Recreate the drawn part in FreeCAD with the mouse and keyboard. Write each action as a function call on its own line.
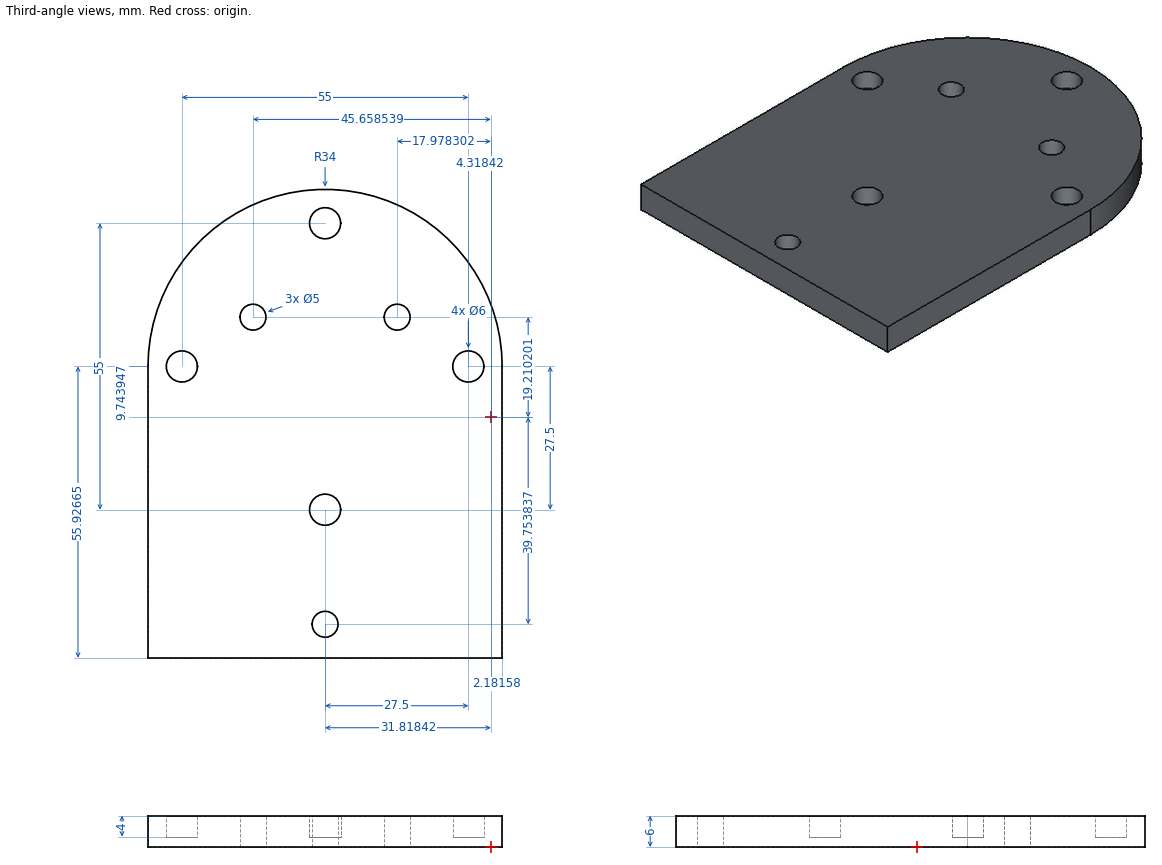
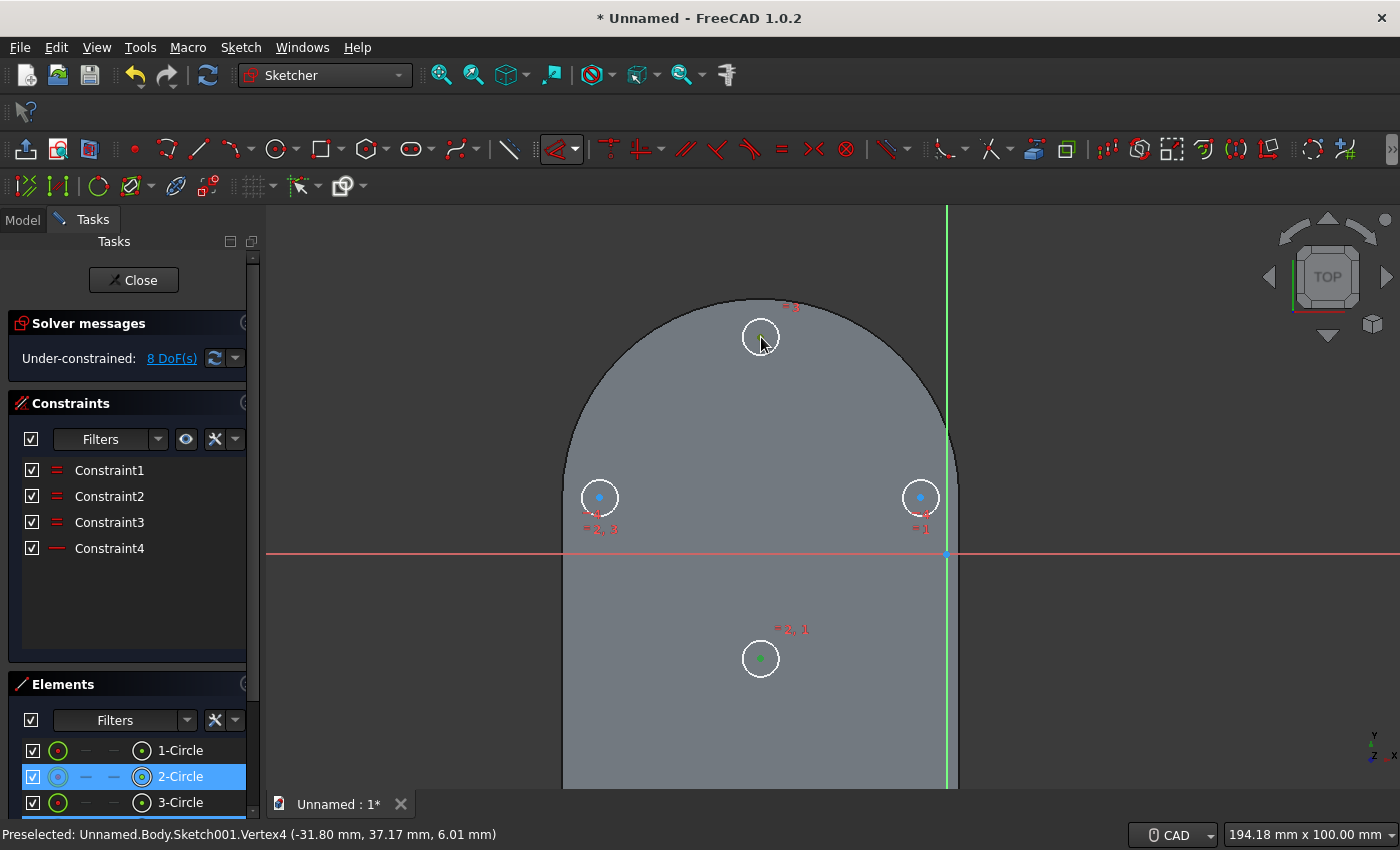
key(v)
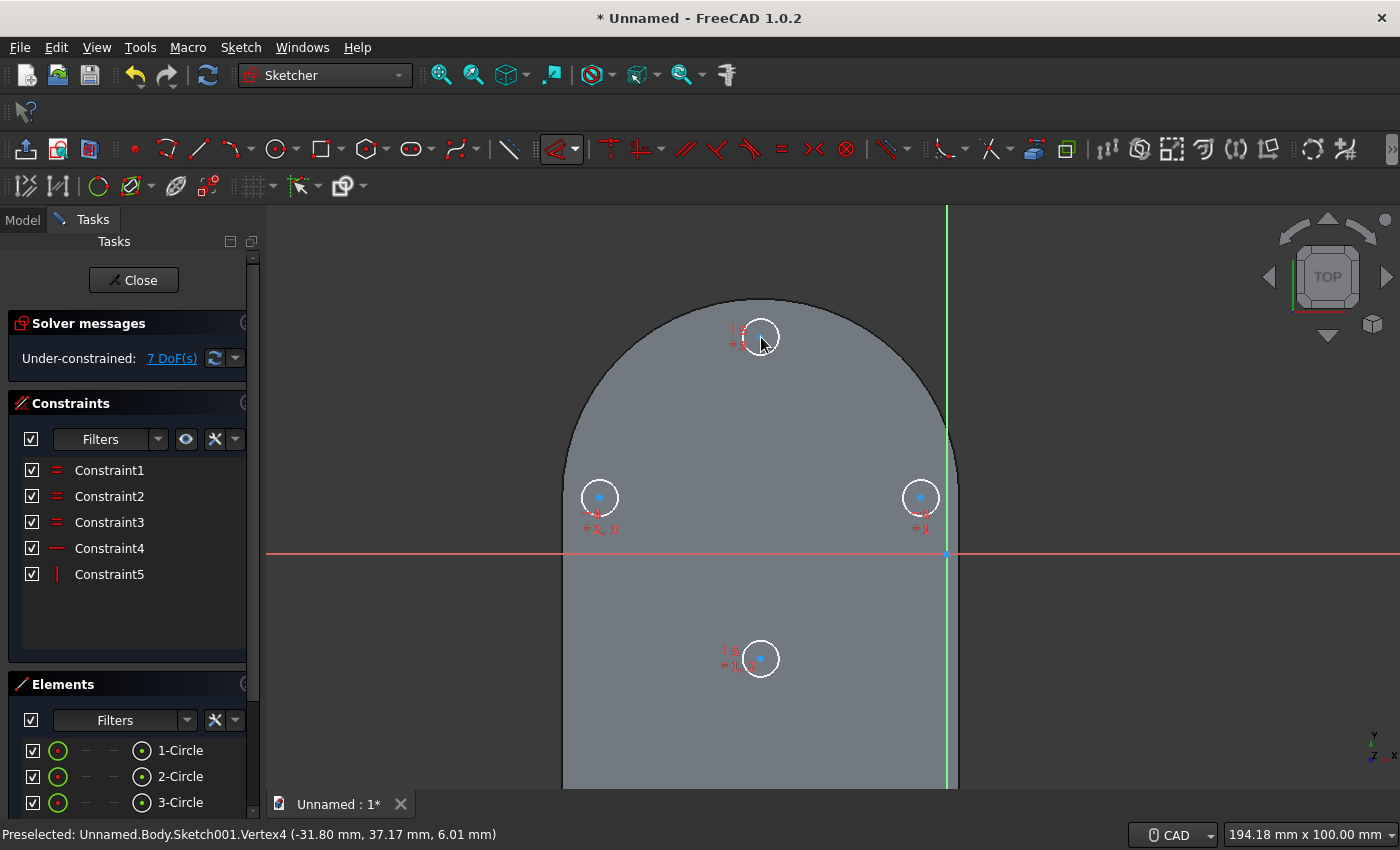
click(934, 485)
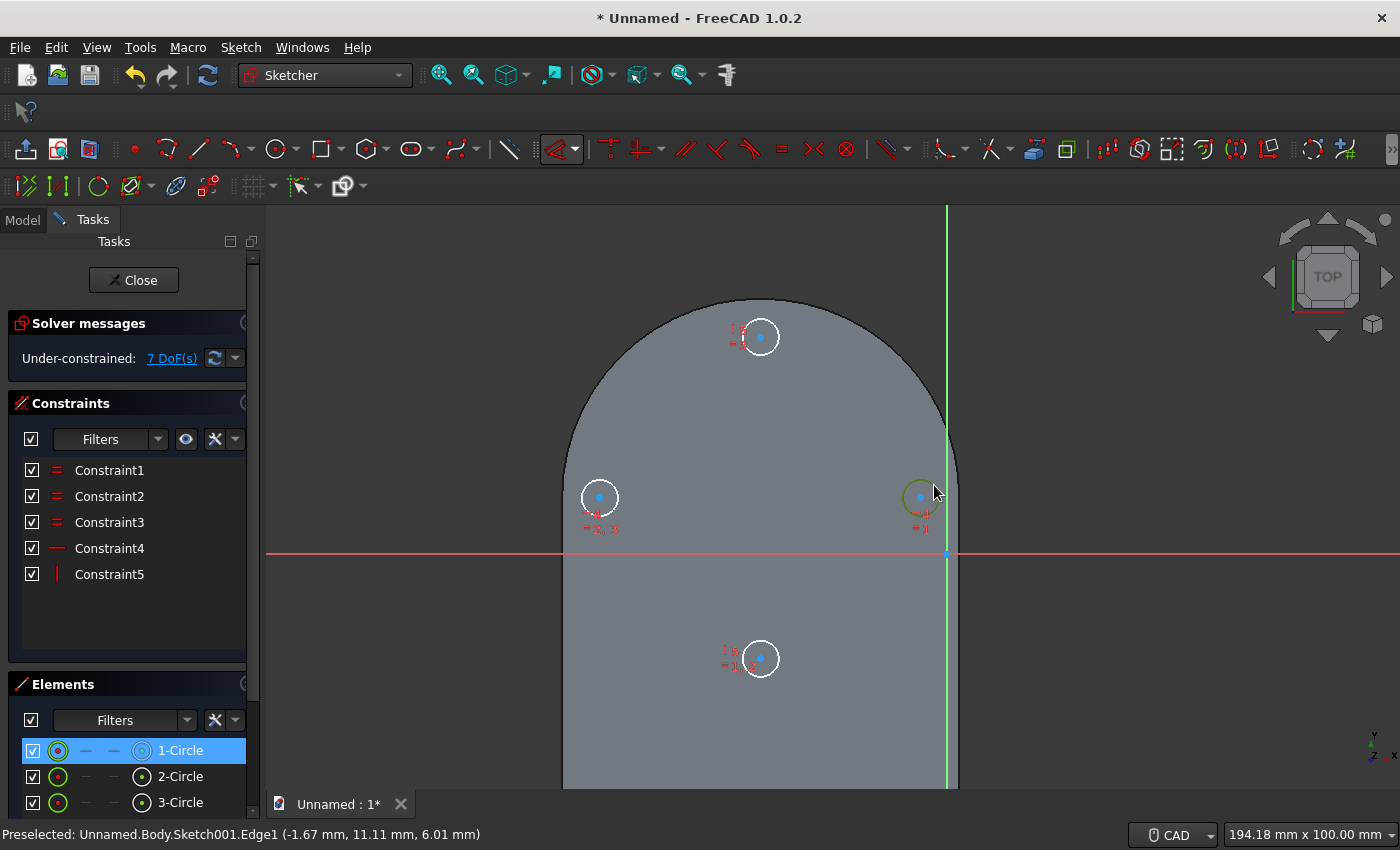
key(k)
key(o)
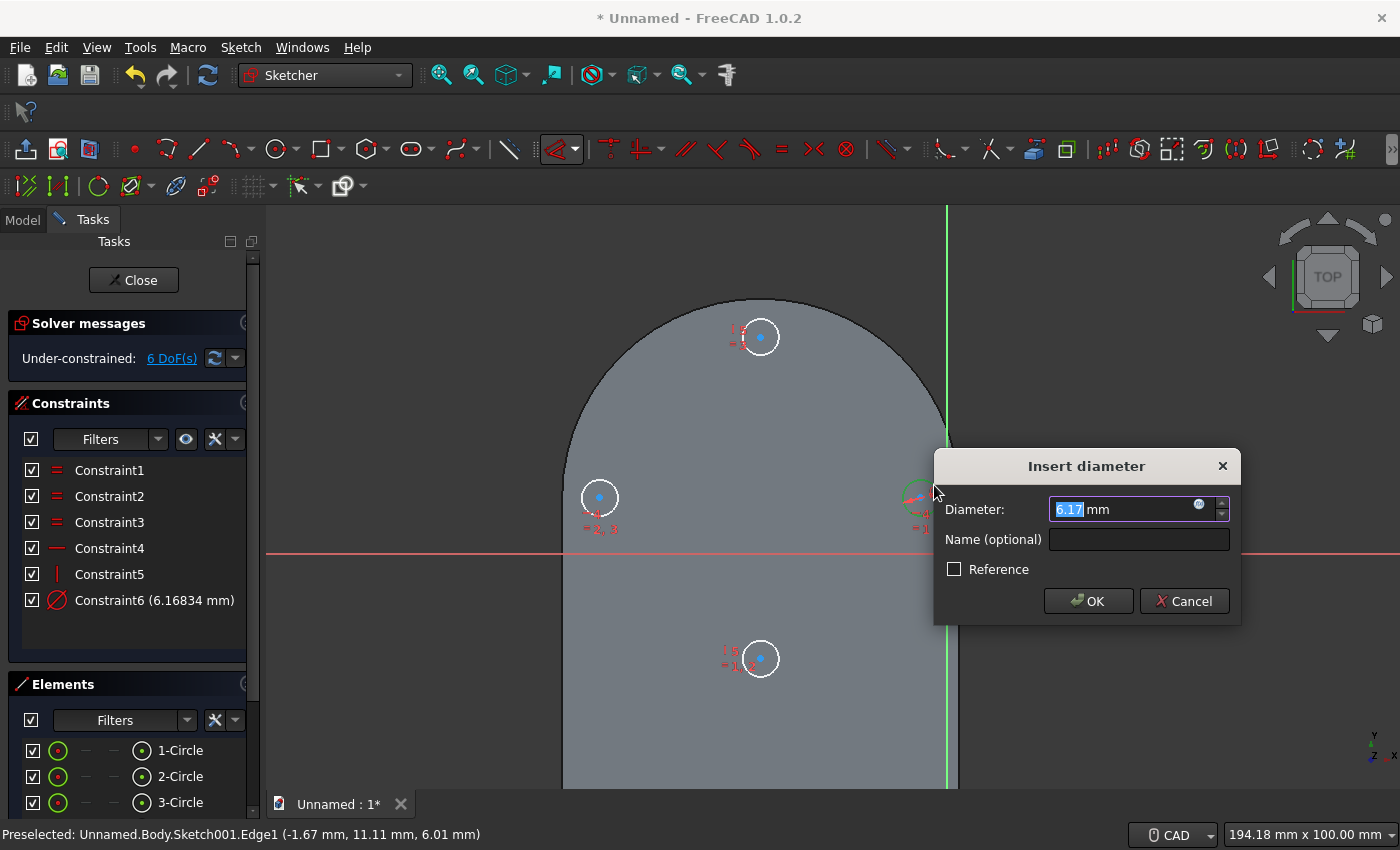
text(6)
key(Return)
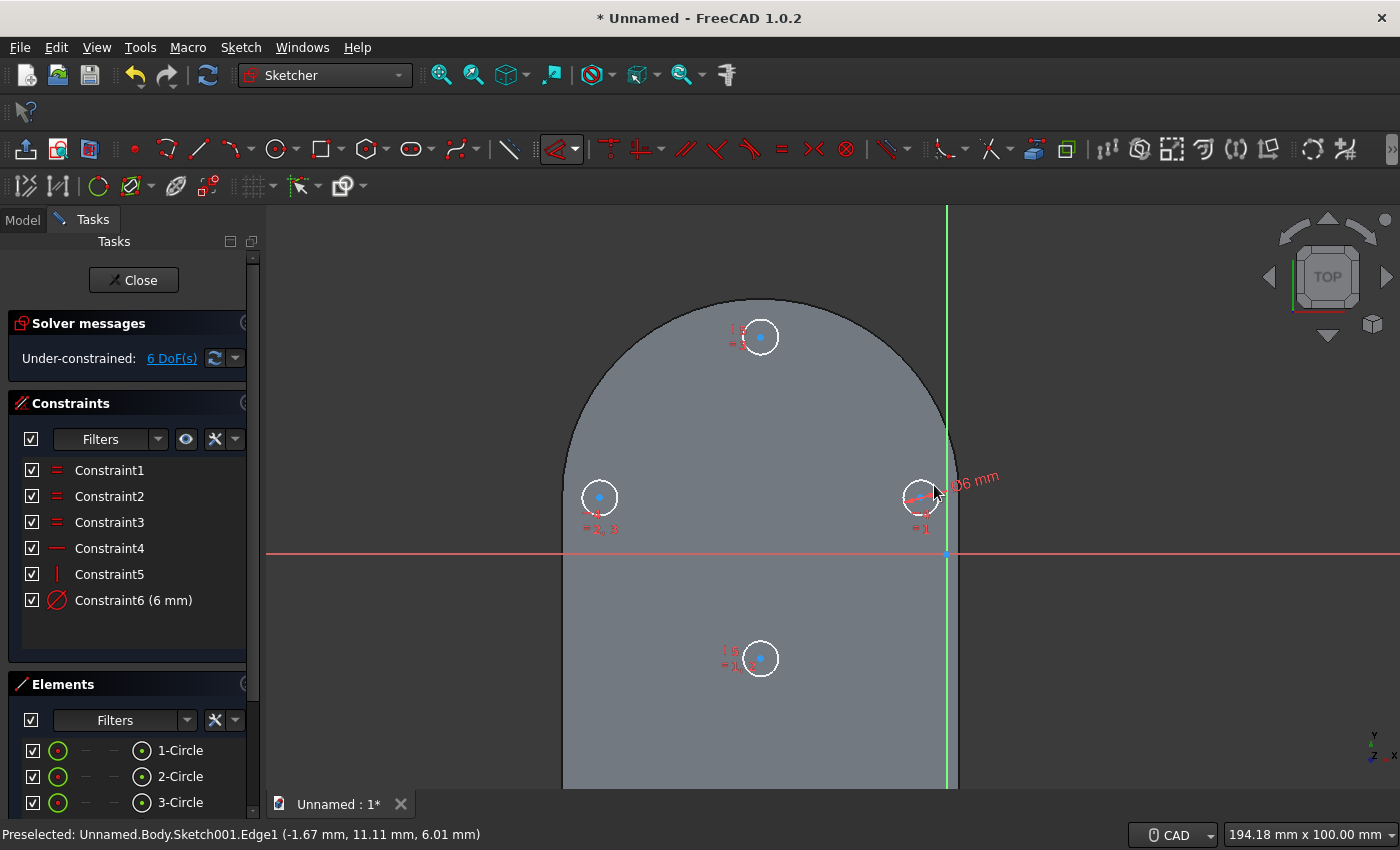
click(921, 498)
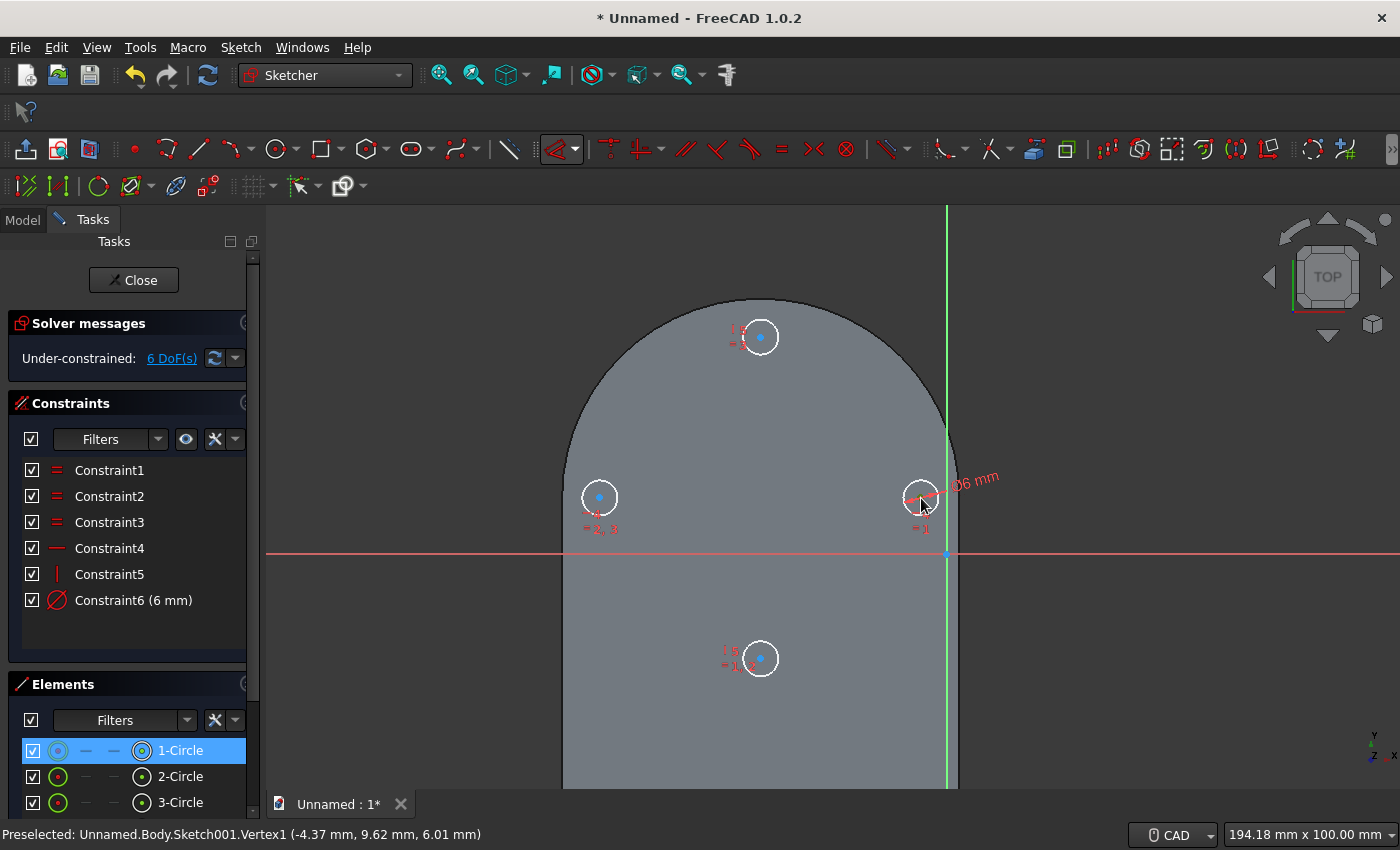
click(600, 498)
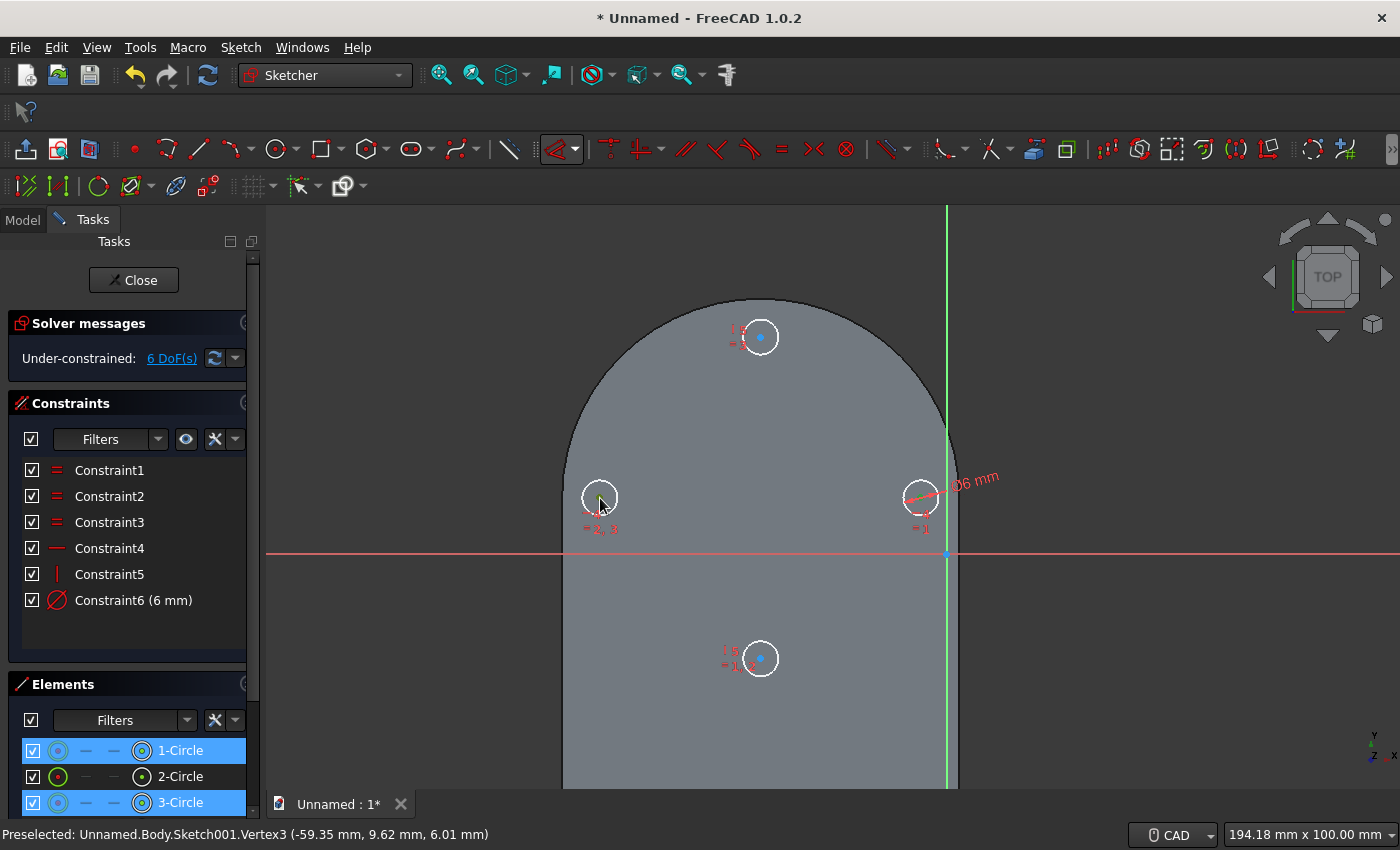
key(l)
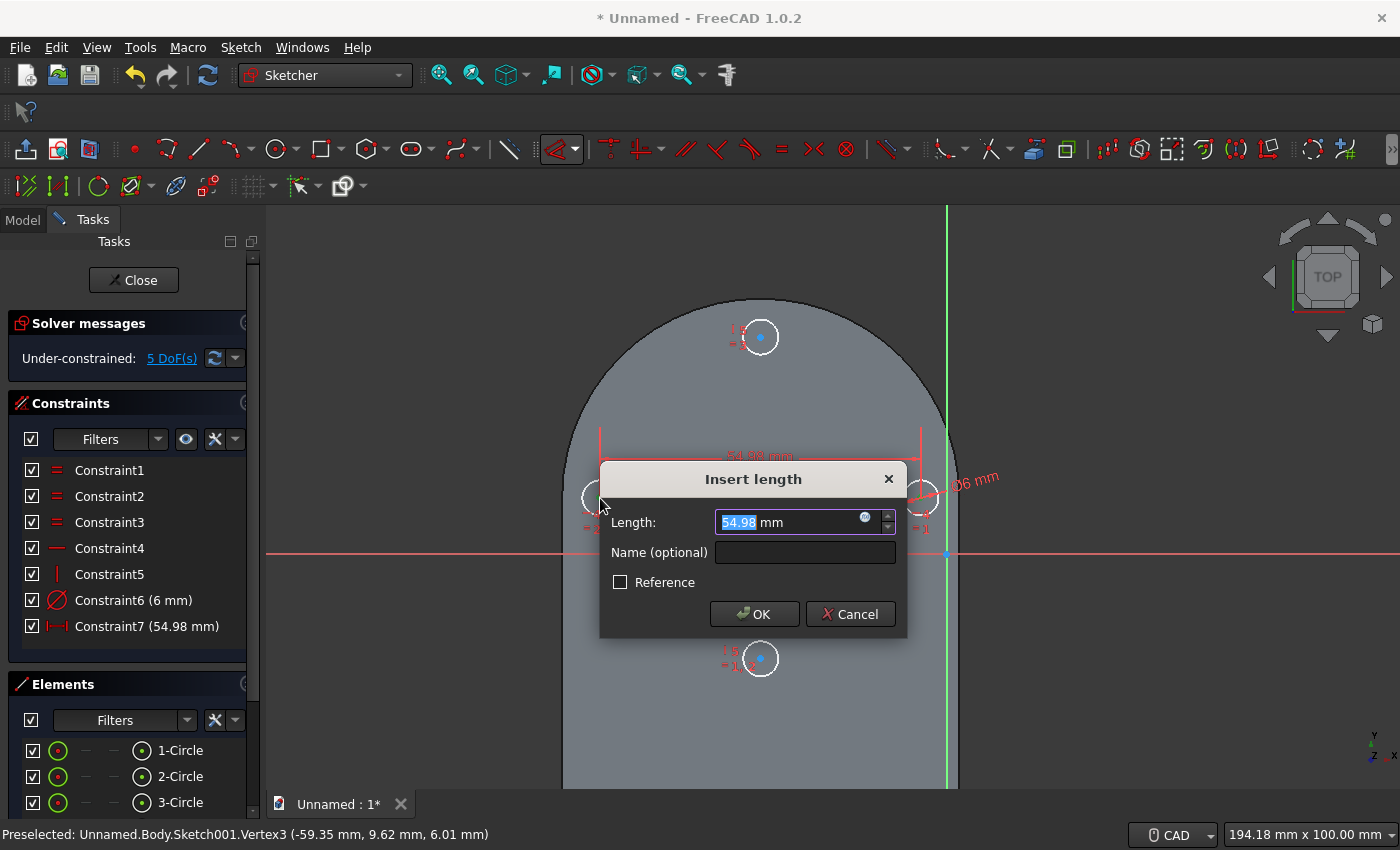
text(55)
key(Return)